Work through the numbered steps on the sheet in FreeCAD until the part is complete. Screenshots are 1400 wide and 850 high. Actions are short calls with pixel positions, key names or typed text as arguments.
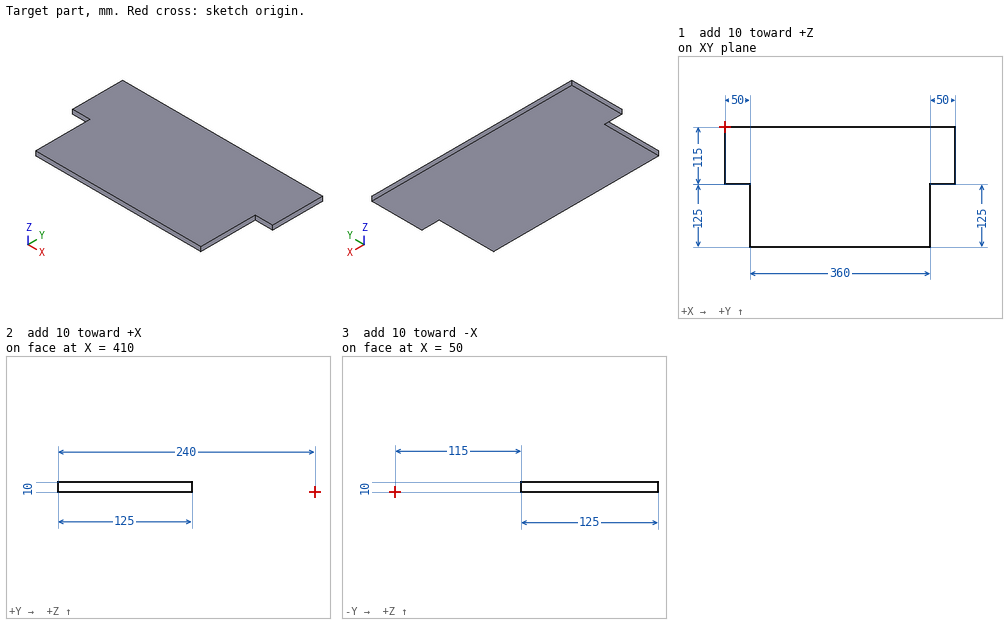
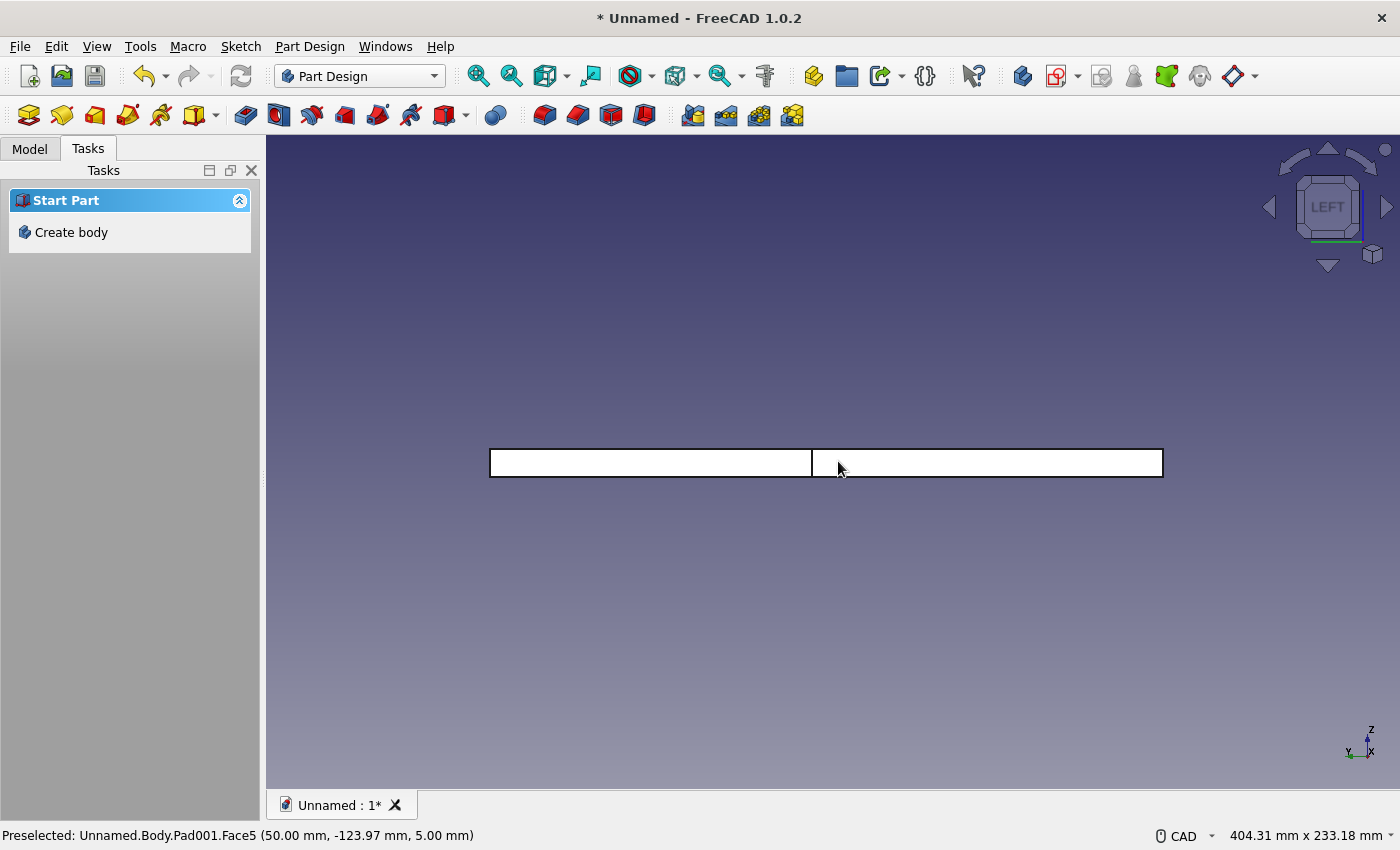
click(837, 462)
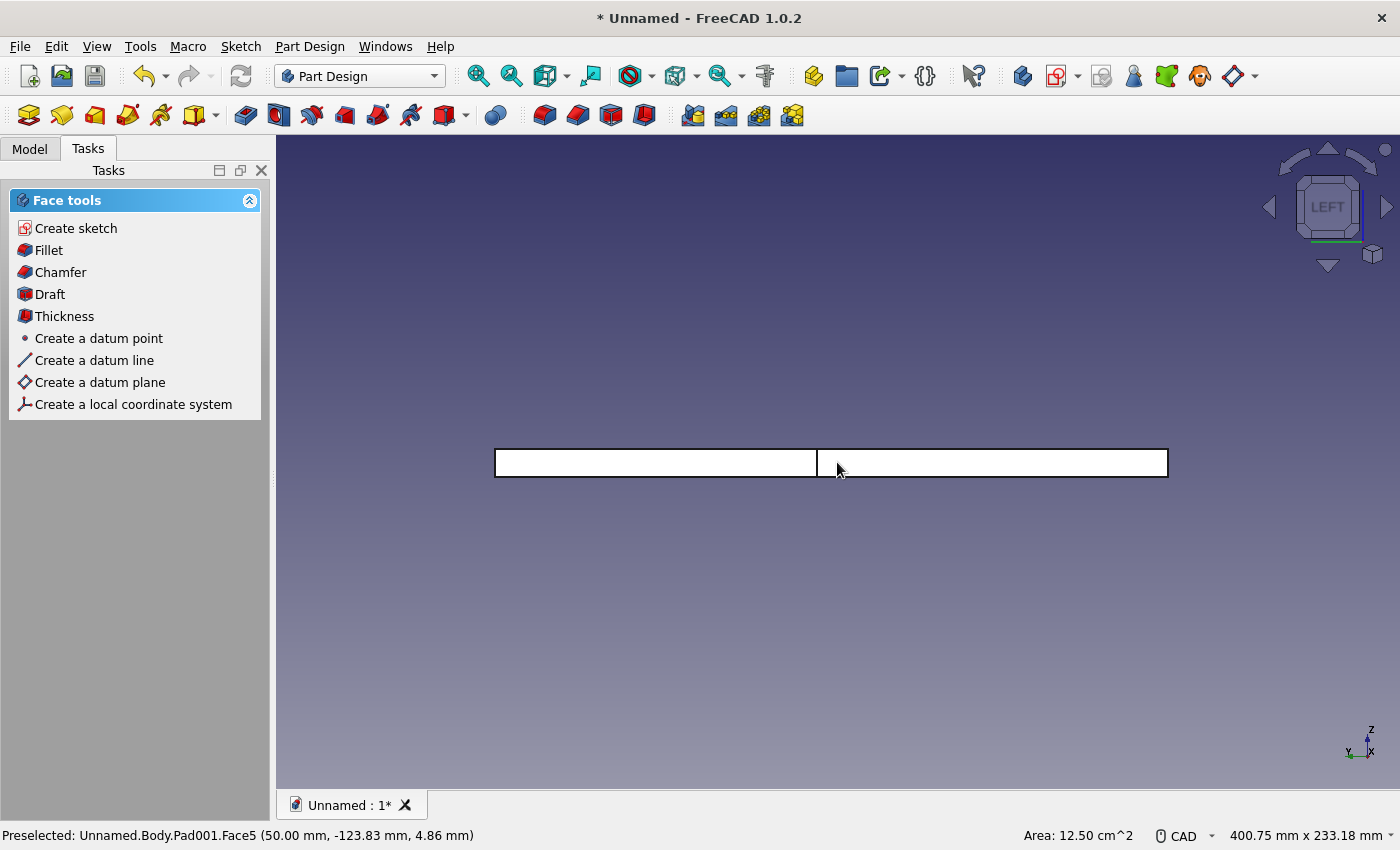
click(1056, 76)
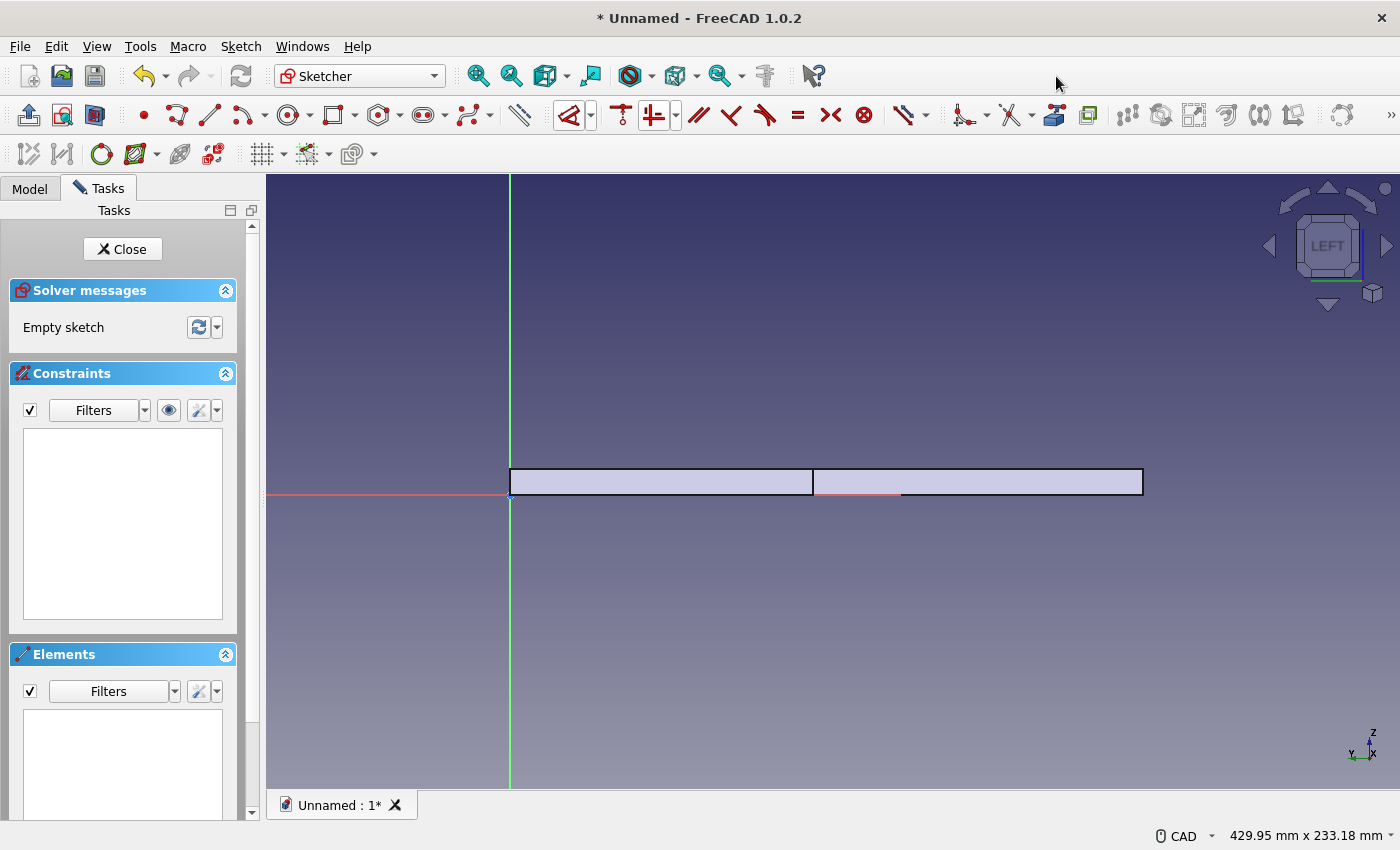
click(95, 116)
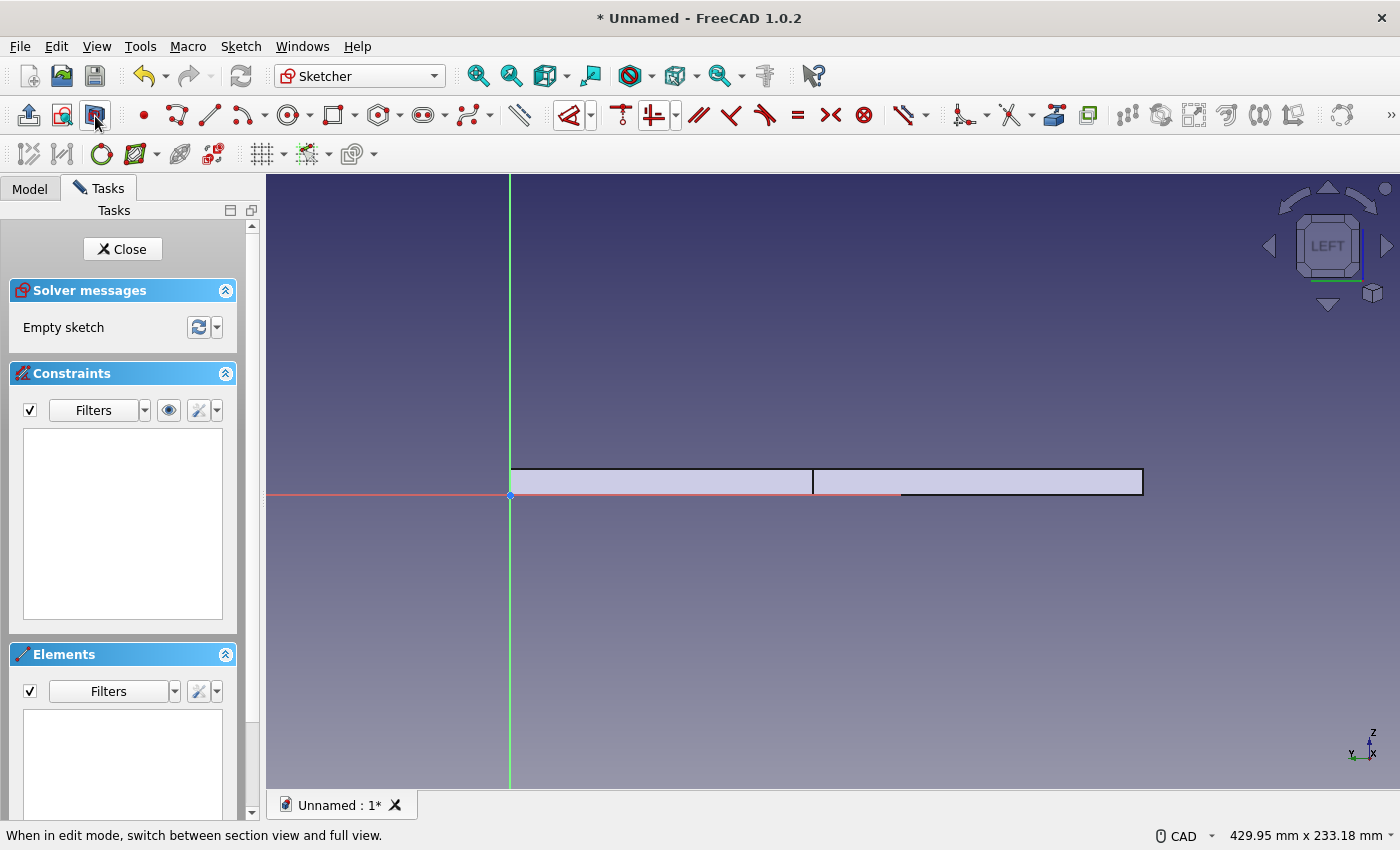
click(332, 116)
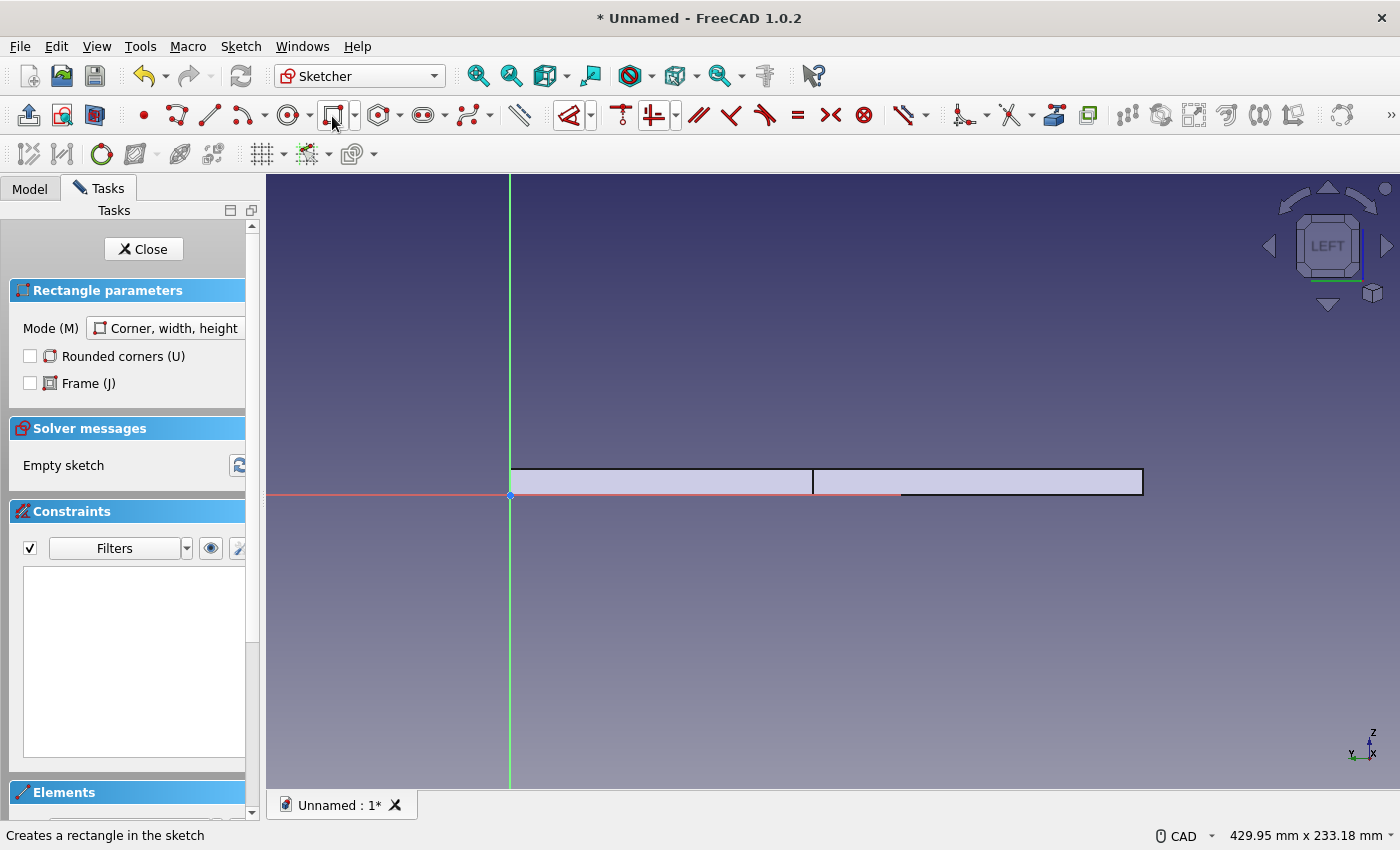
click(813, 469)
click(1143, 495)
key(Escape)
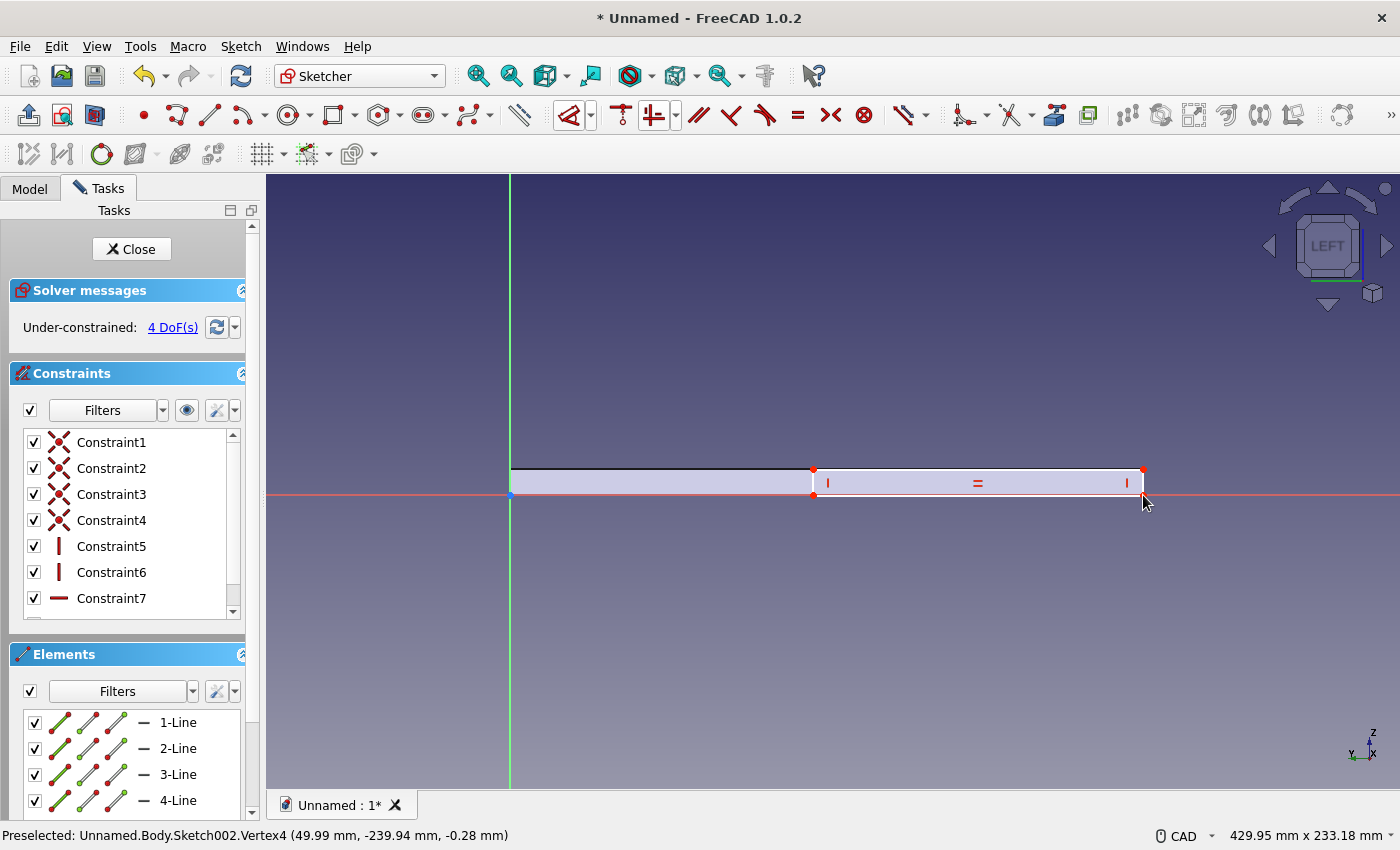
click(813, 496)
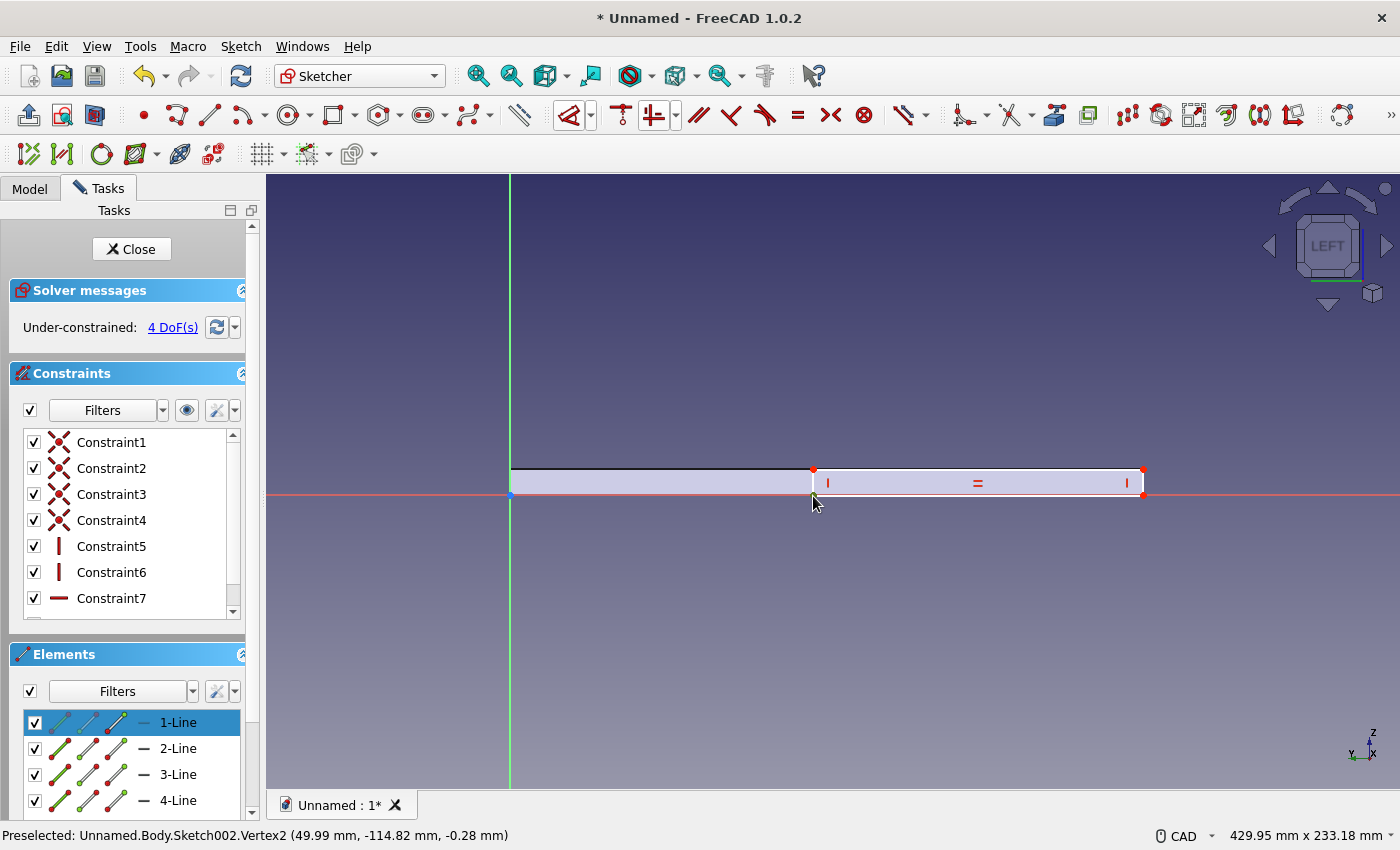
click(361, 495)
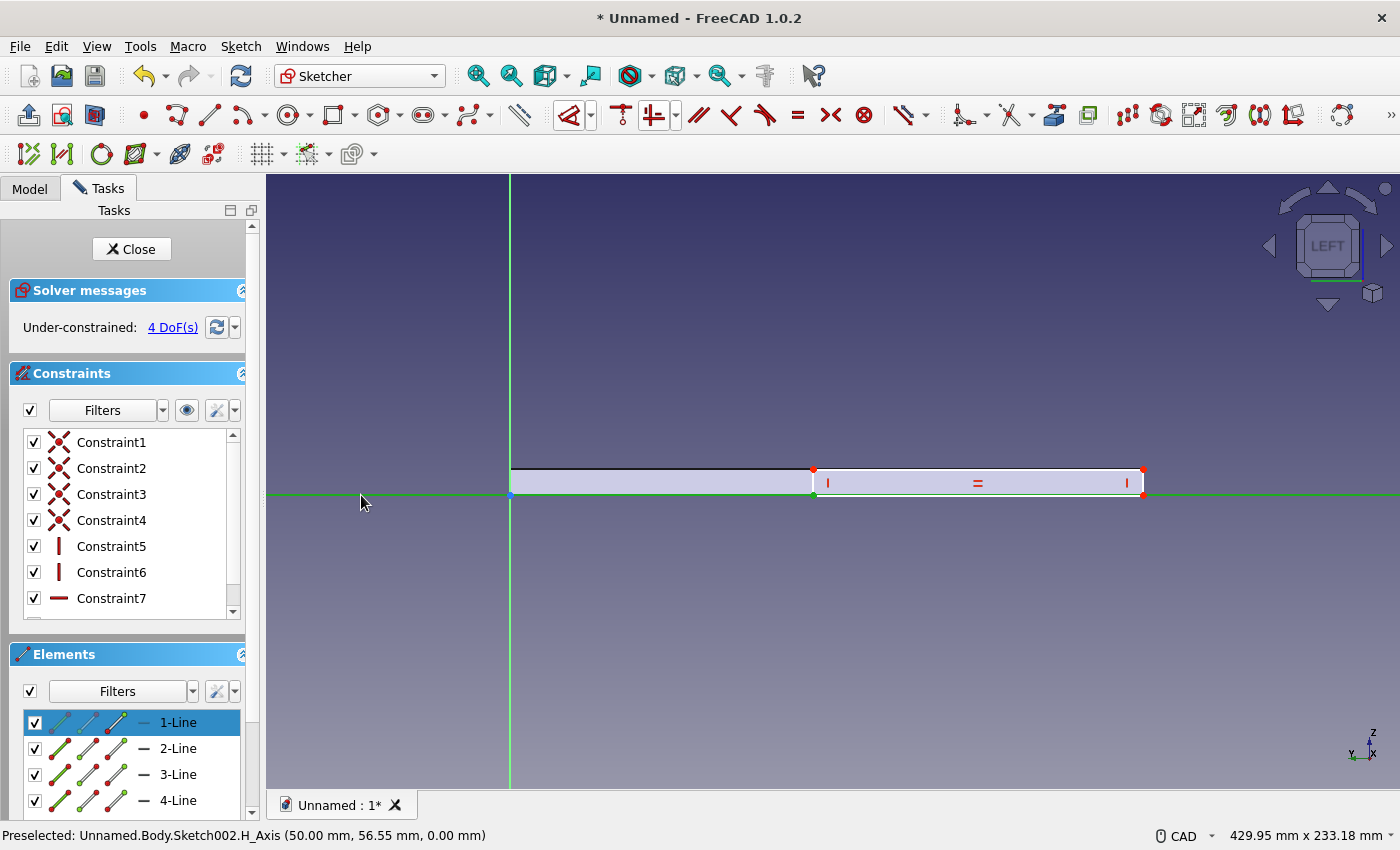
click(621, 116)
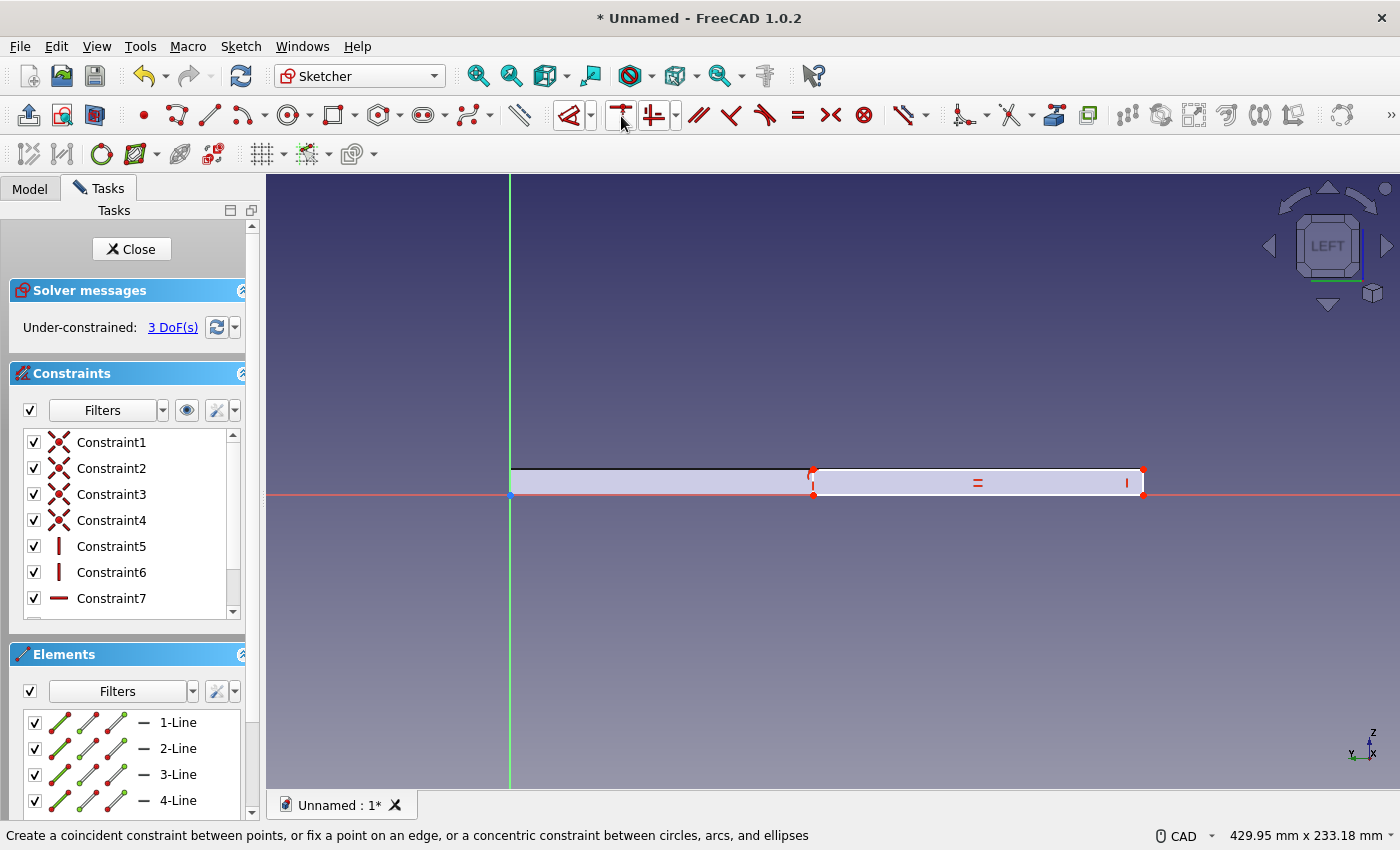
scroll(813, 480, up, 3)